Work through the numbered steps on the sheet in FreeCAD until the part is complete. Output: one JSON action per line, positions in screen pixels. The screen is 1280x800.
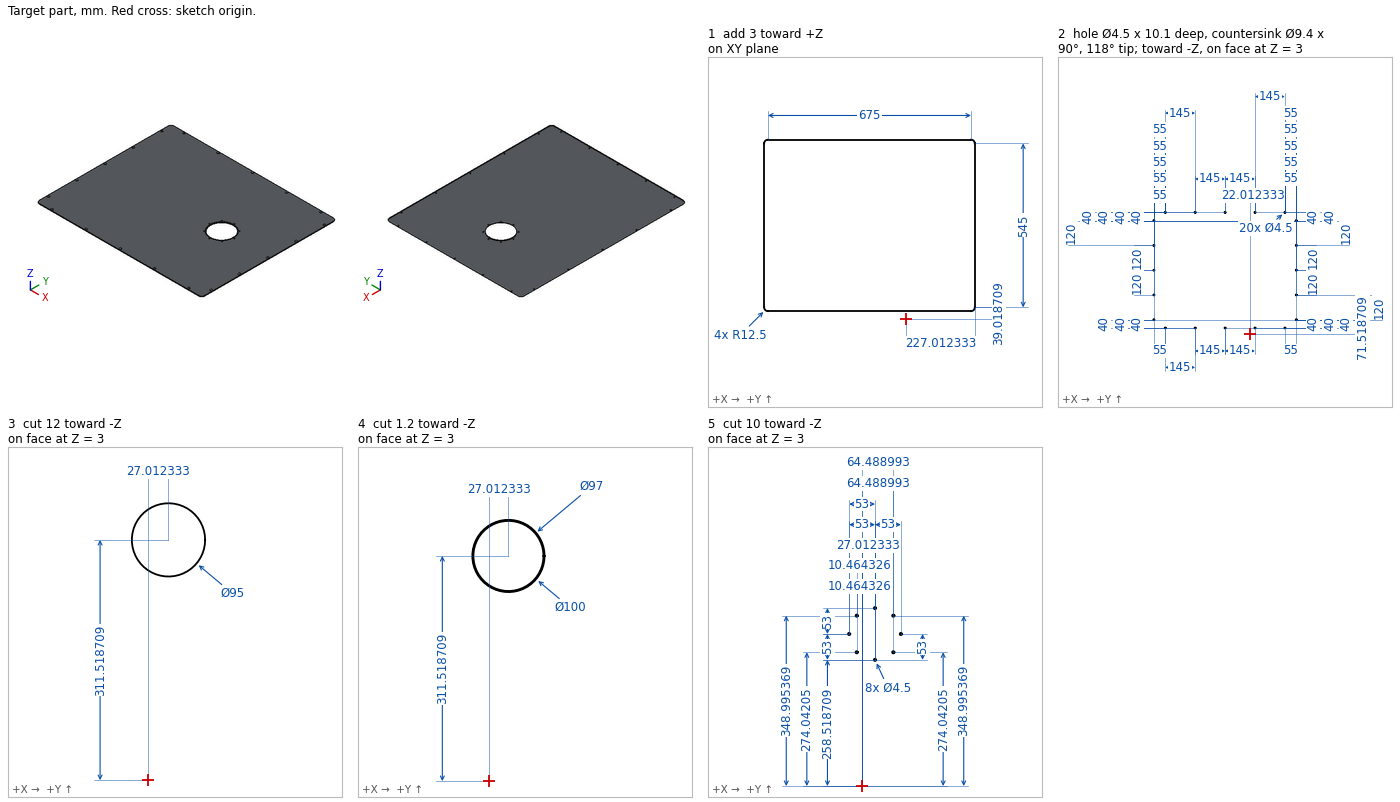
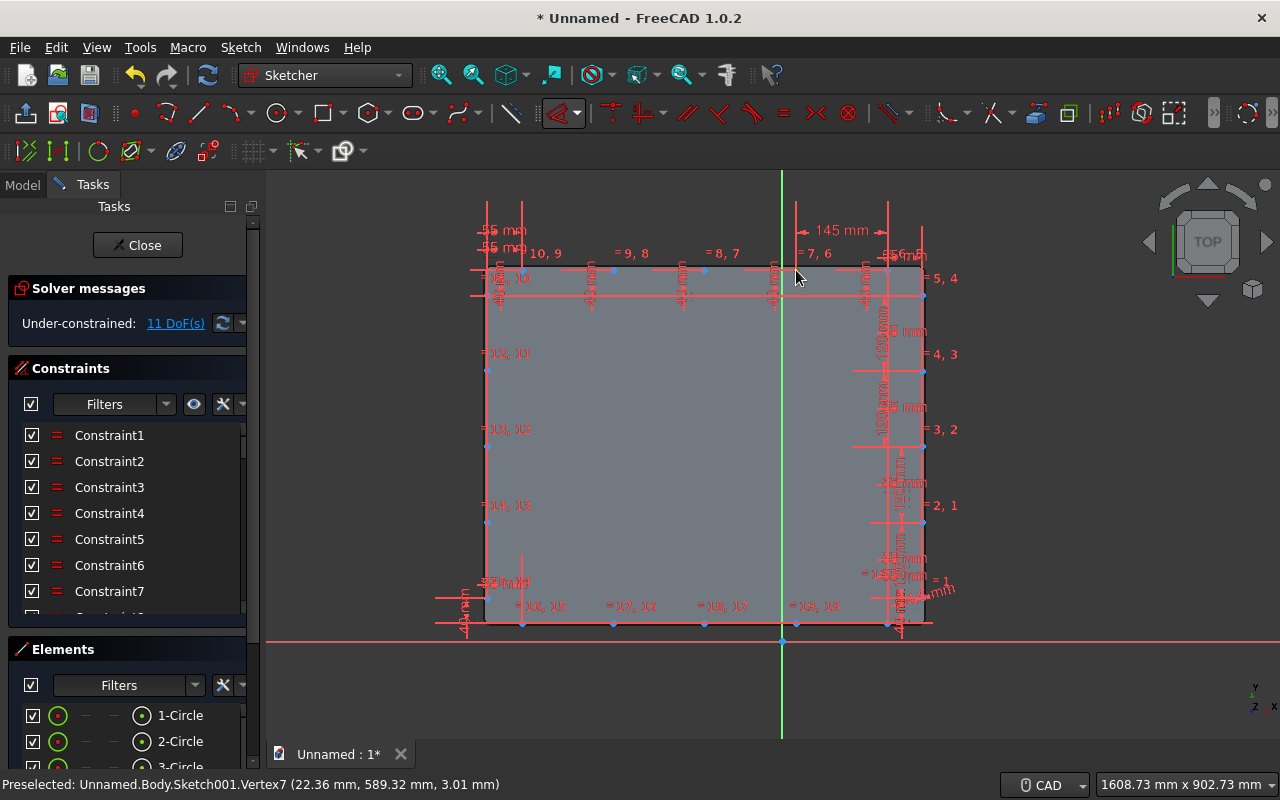
{"action": "left_click", "coordinate": [704, 270]}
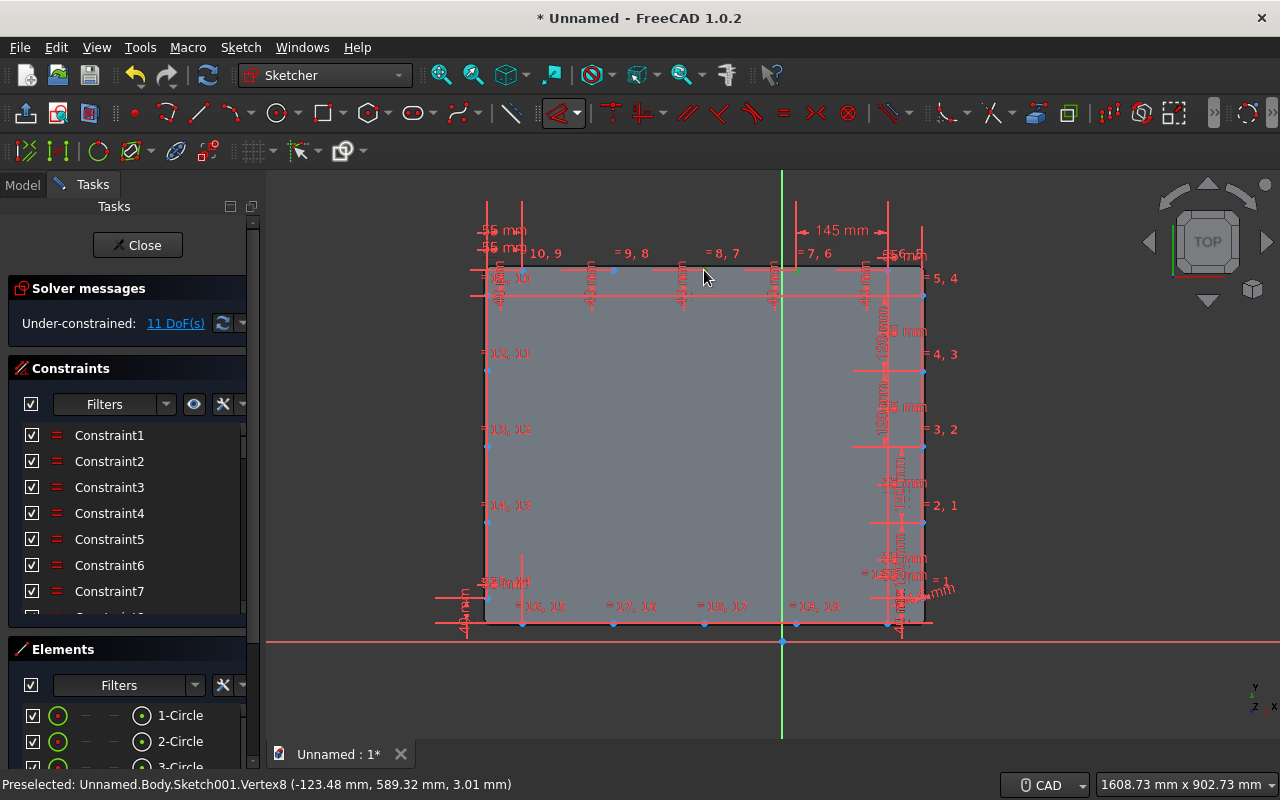
{"action": "left_click", "coordinate": [580, 114]}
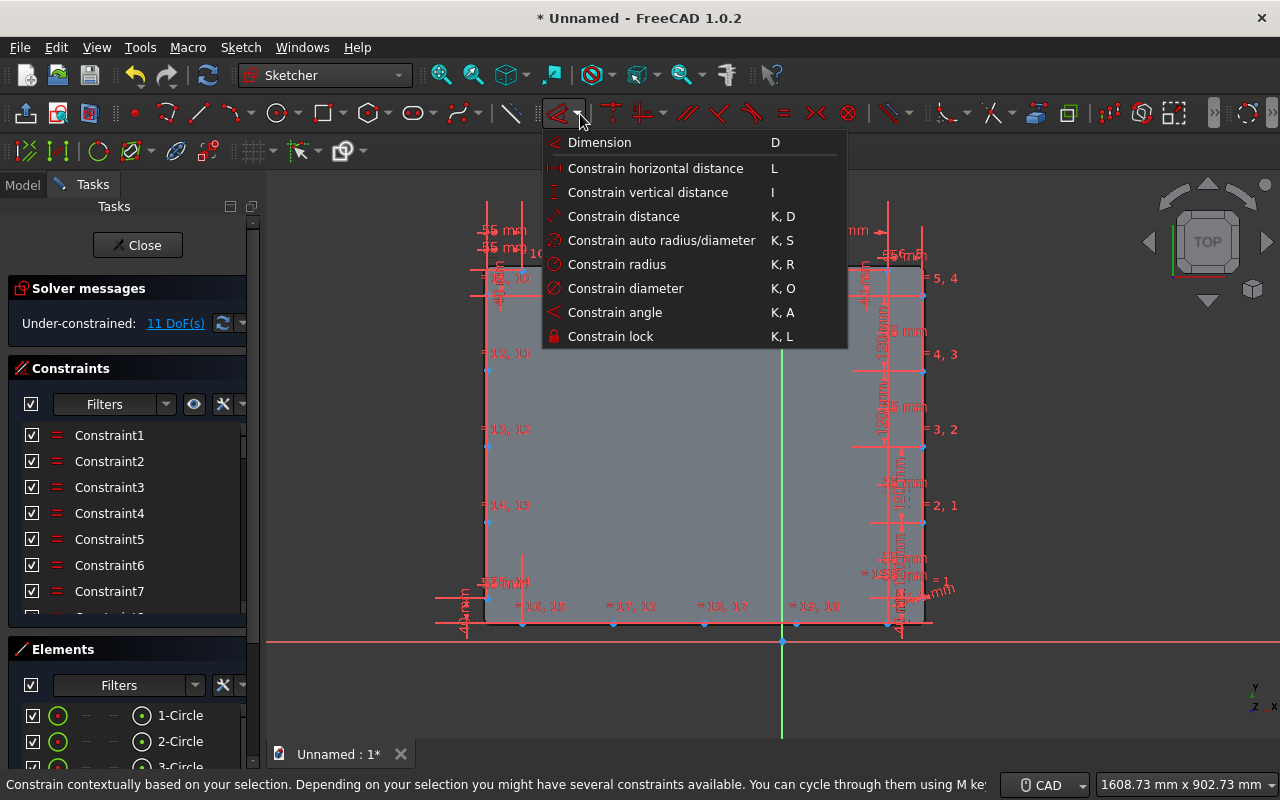
{"action": "left_click", "coordinate": [695, 168]}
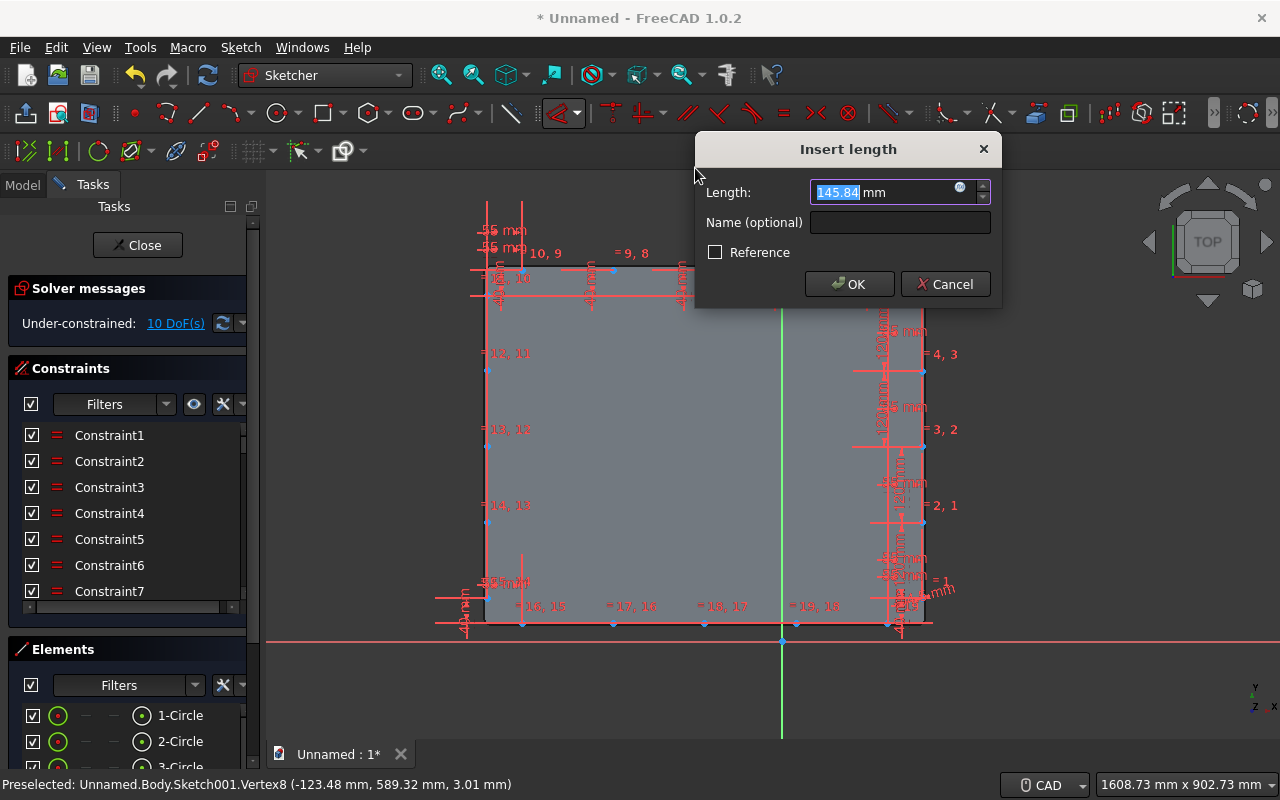
{"action": "type", "text": "145"}
{"action": "key", "text": "Return"}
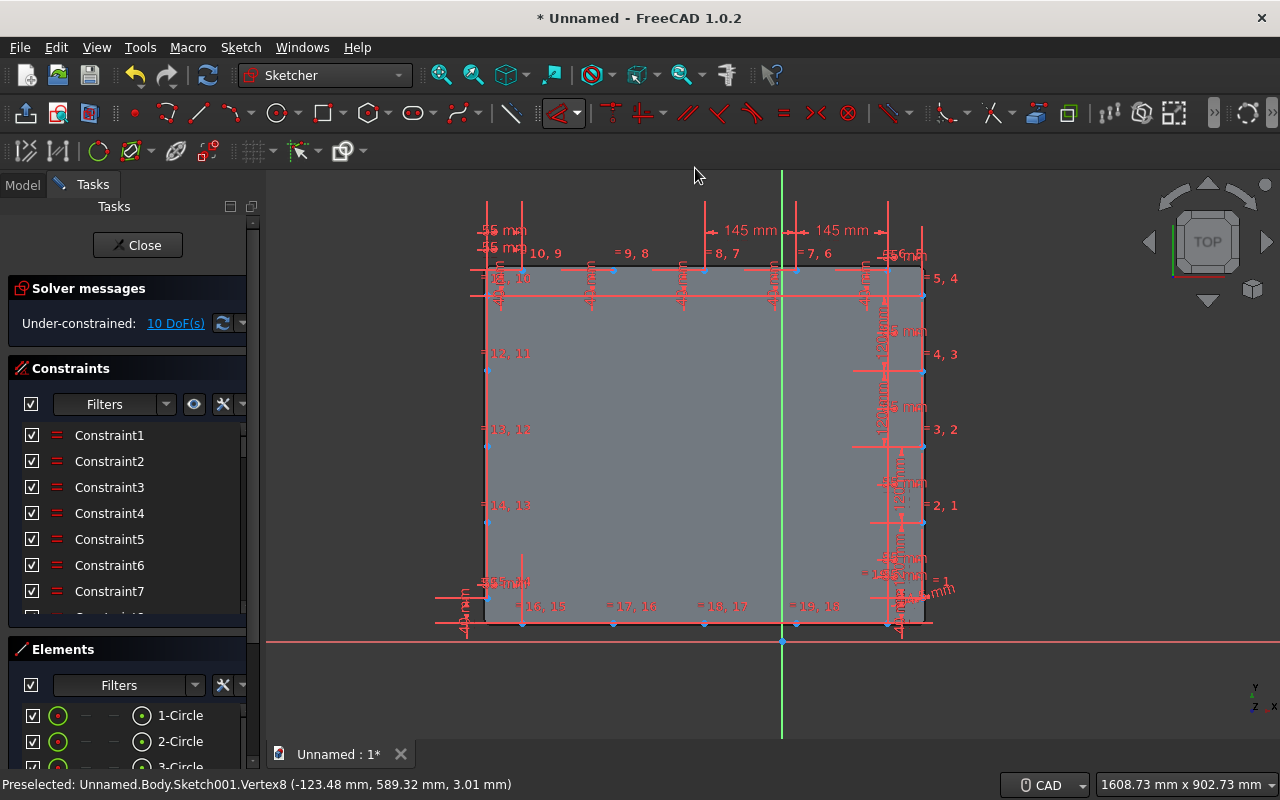
{"action": "left_click", "coordinate": [705, 270]}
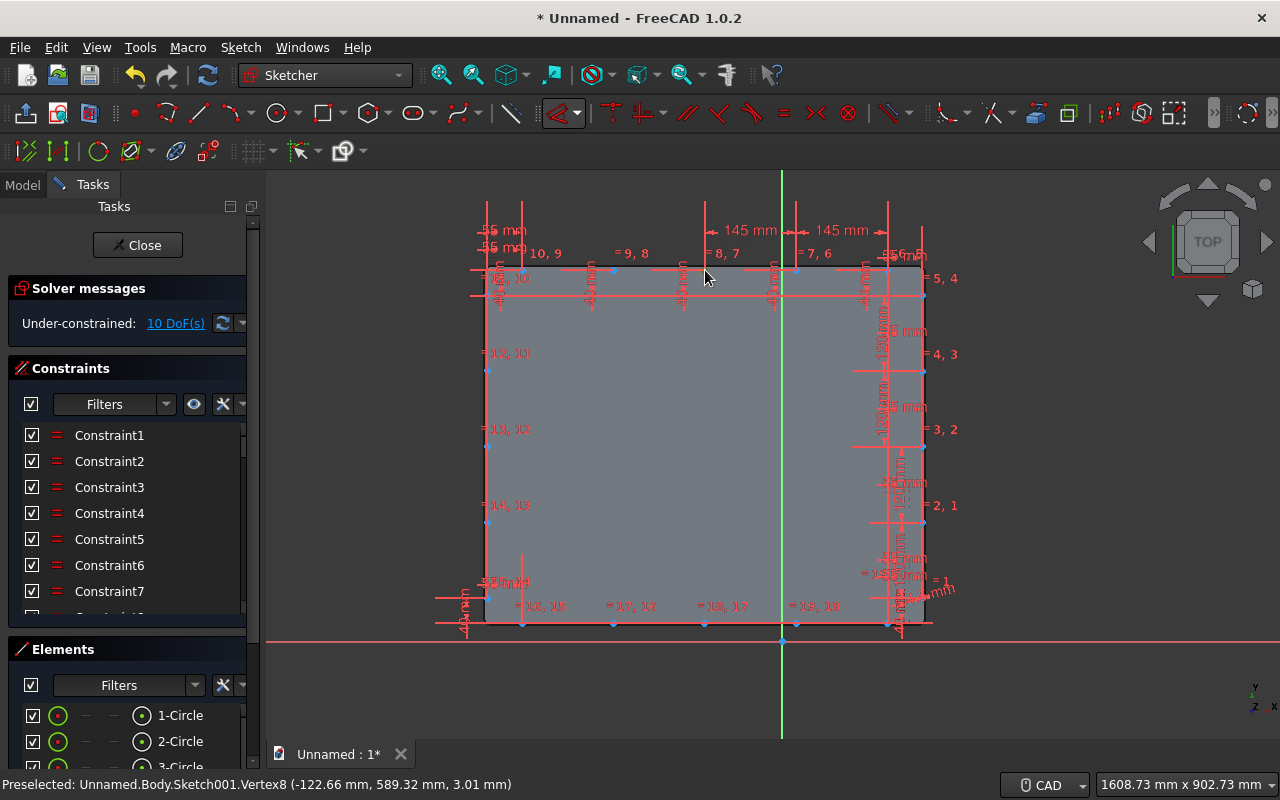
{"action": "left_click", "coordinate": [613, 270]}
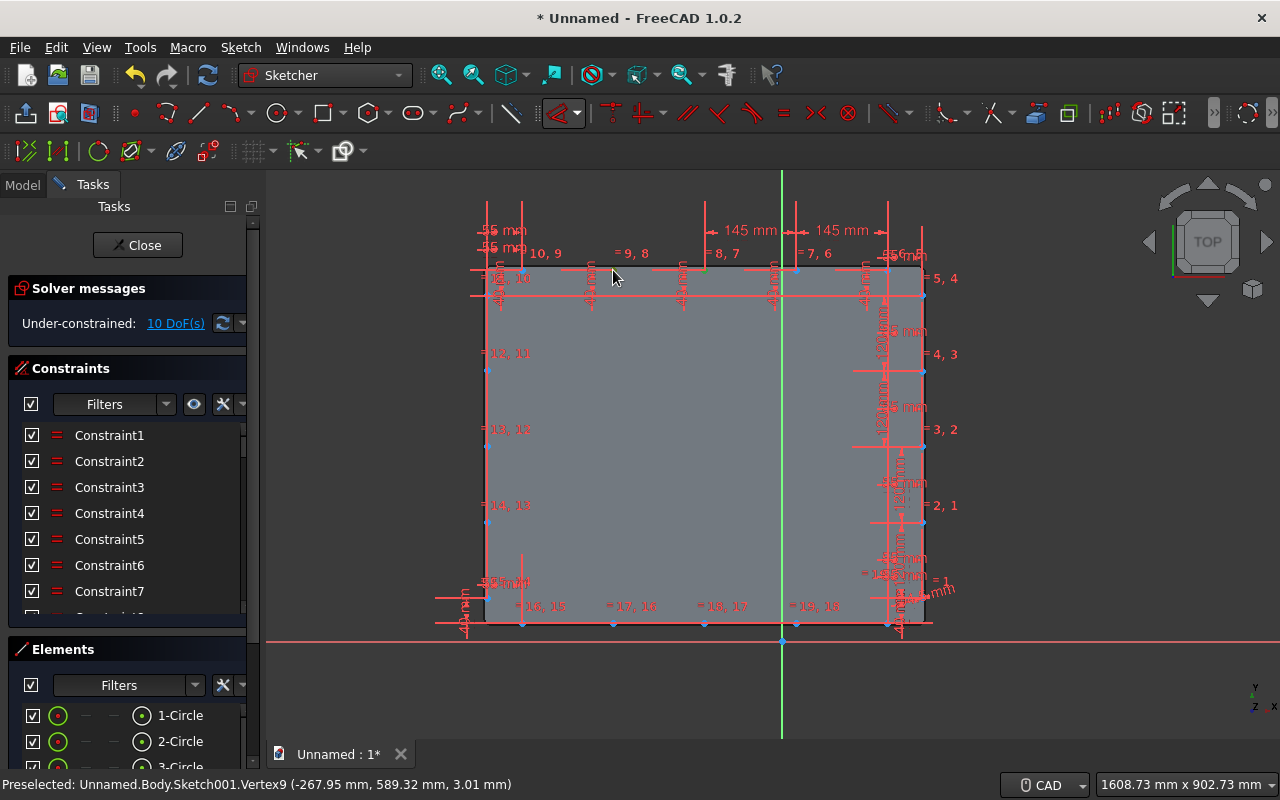
{"action": "key", "text": "l"}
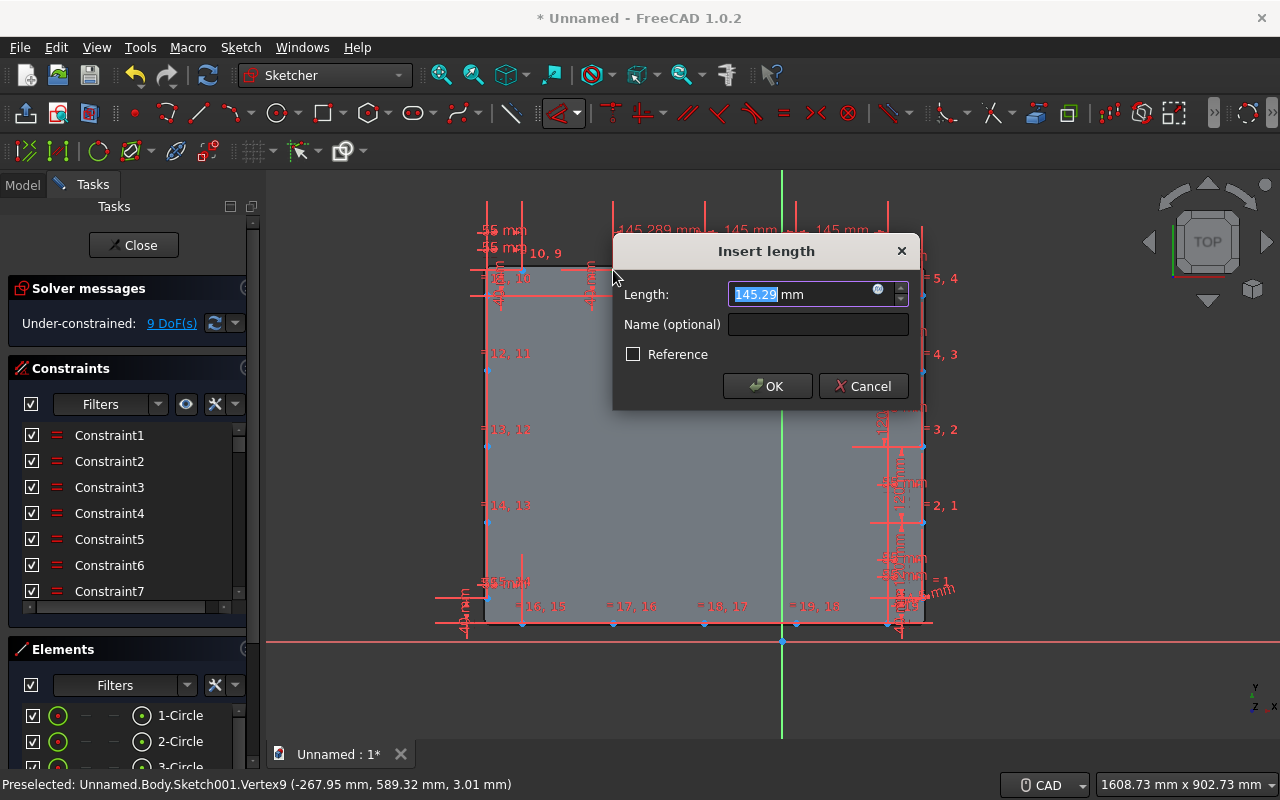
{"action": "type", "text": "145"}
{"action": "key", "text": "Return"}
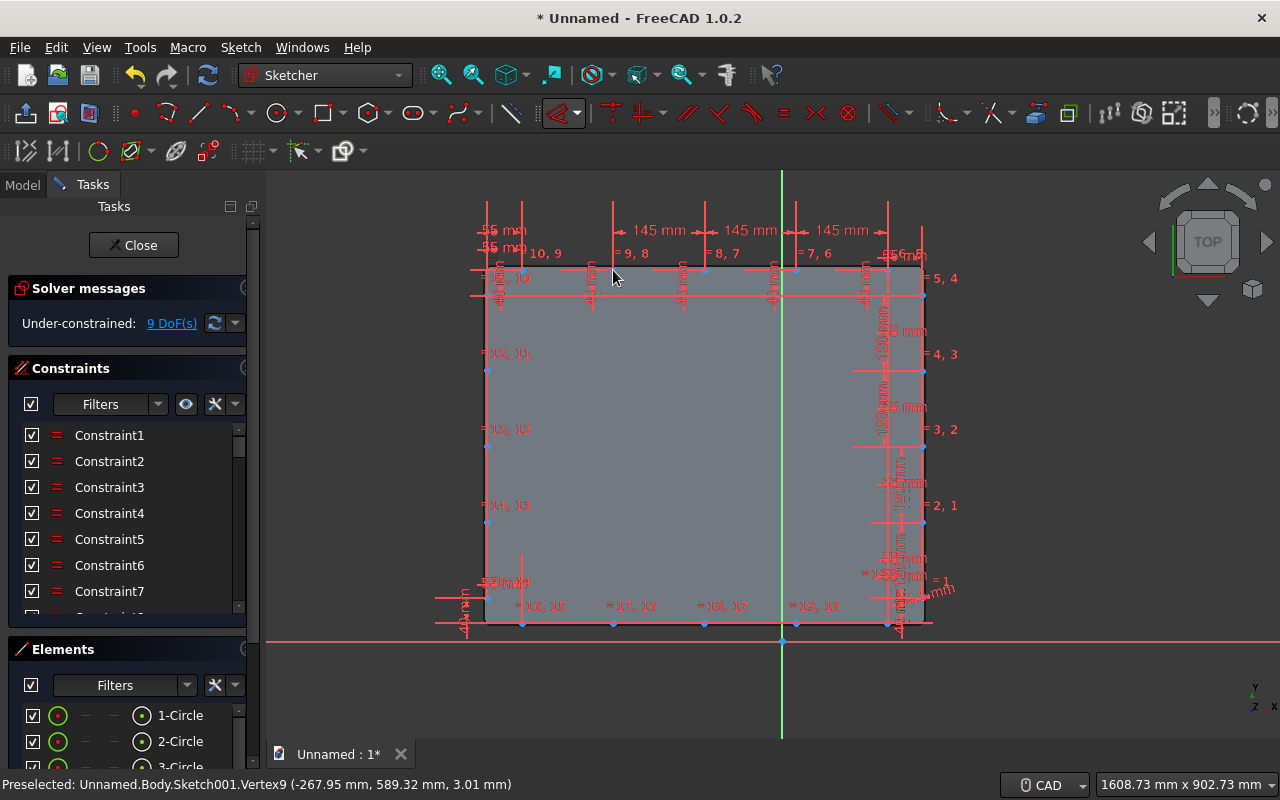
{"action": "left_click", "coordinate": [613, 270]}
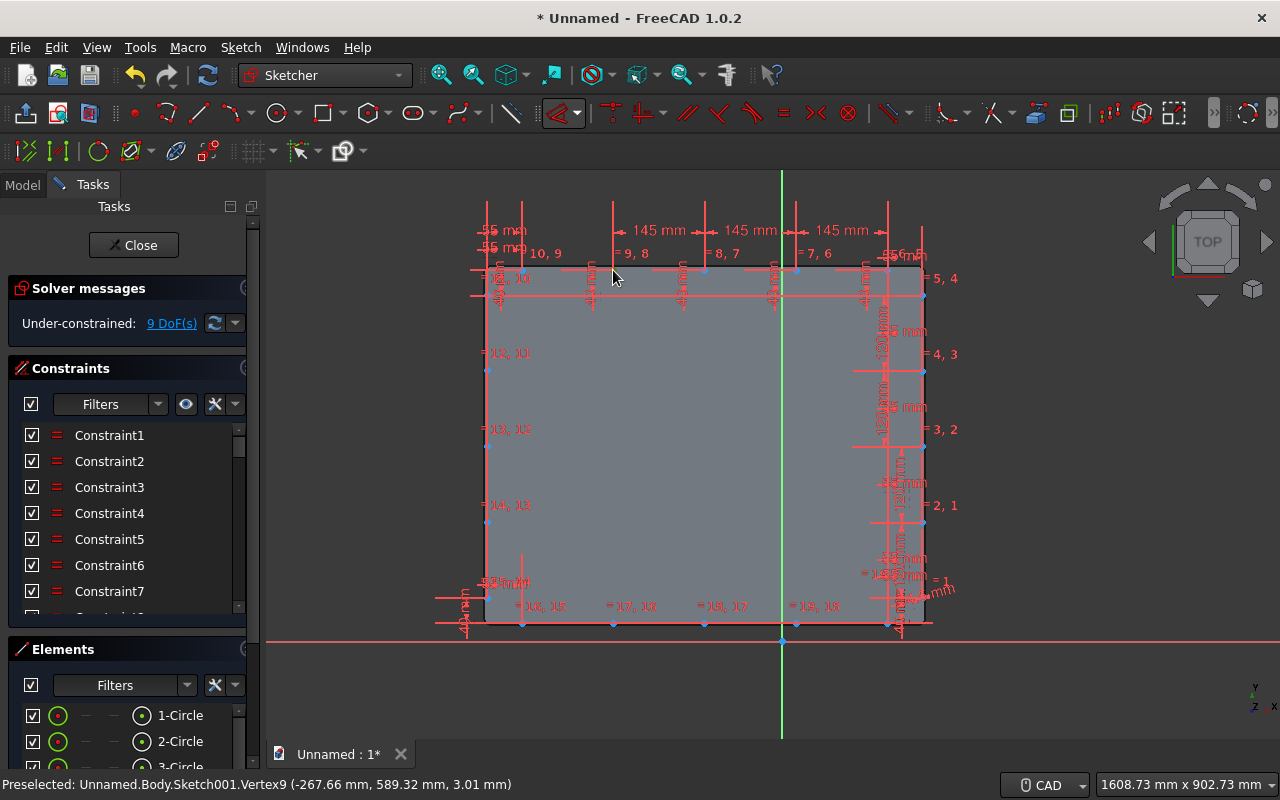
{"action": "left_click", "coordinate": [522, 270]}